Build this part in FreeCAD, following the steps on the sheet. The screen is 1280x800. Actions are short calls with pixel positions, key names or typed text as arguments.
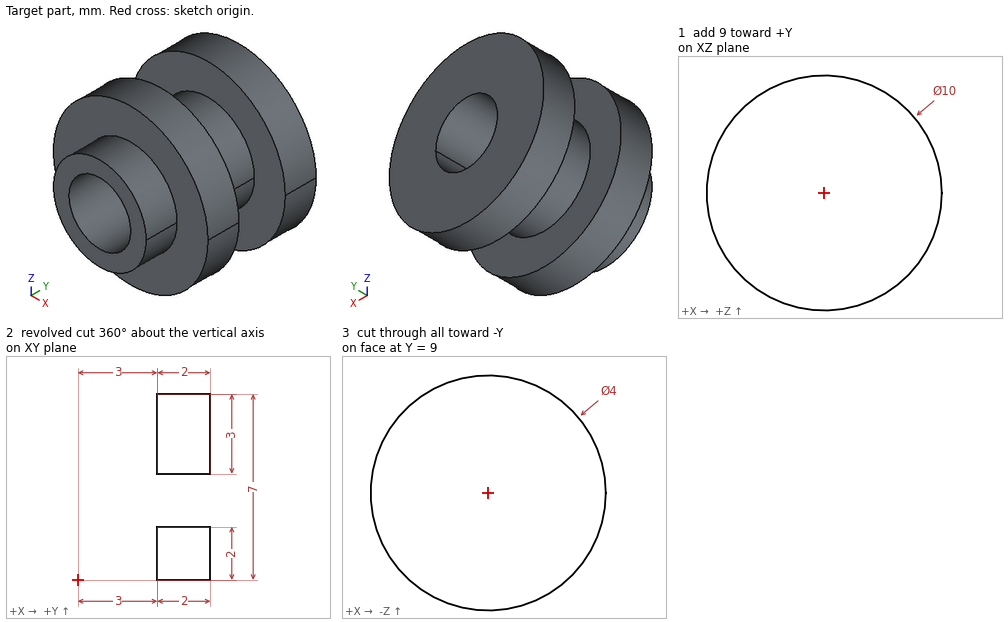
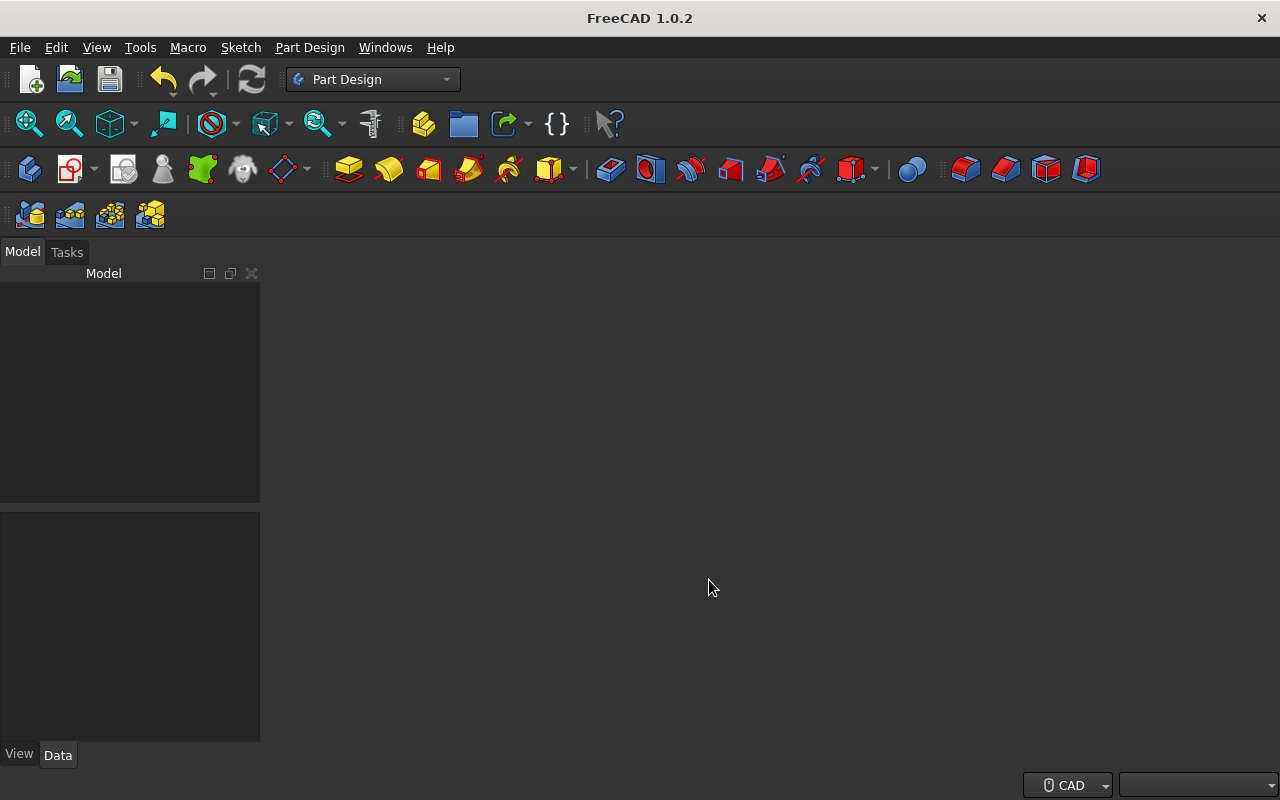
click(30, 80)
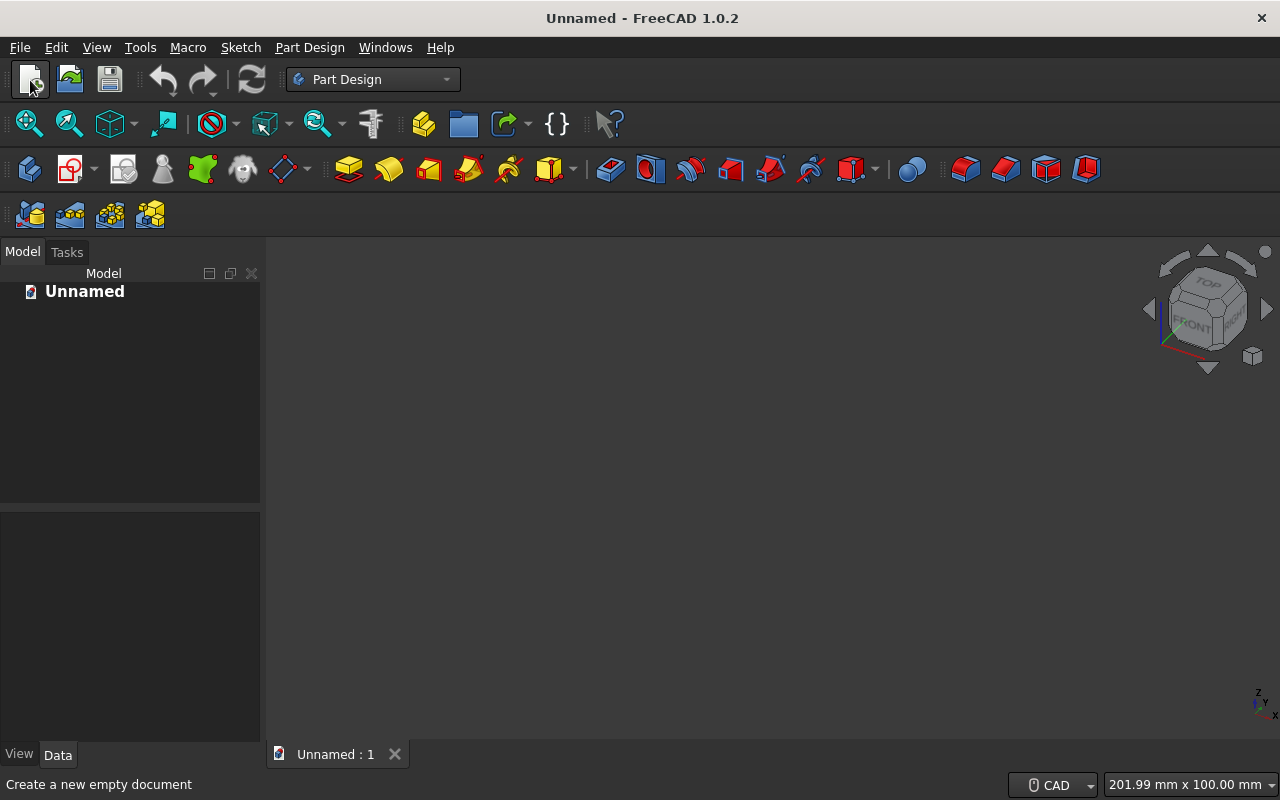
click(70, 170)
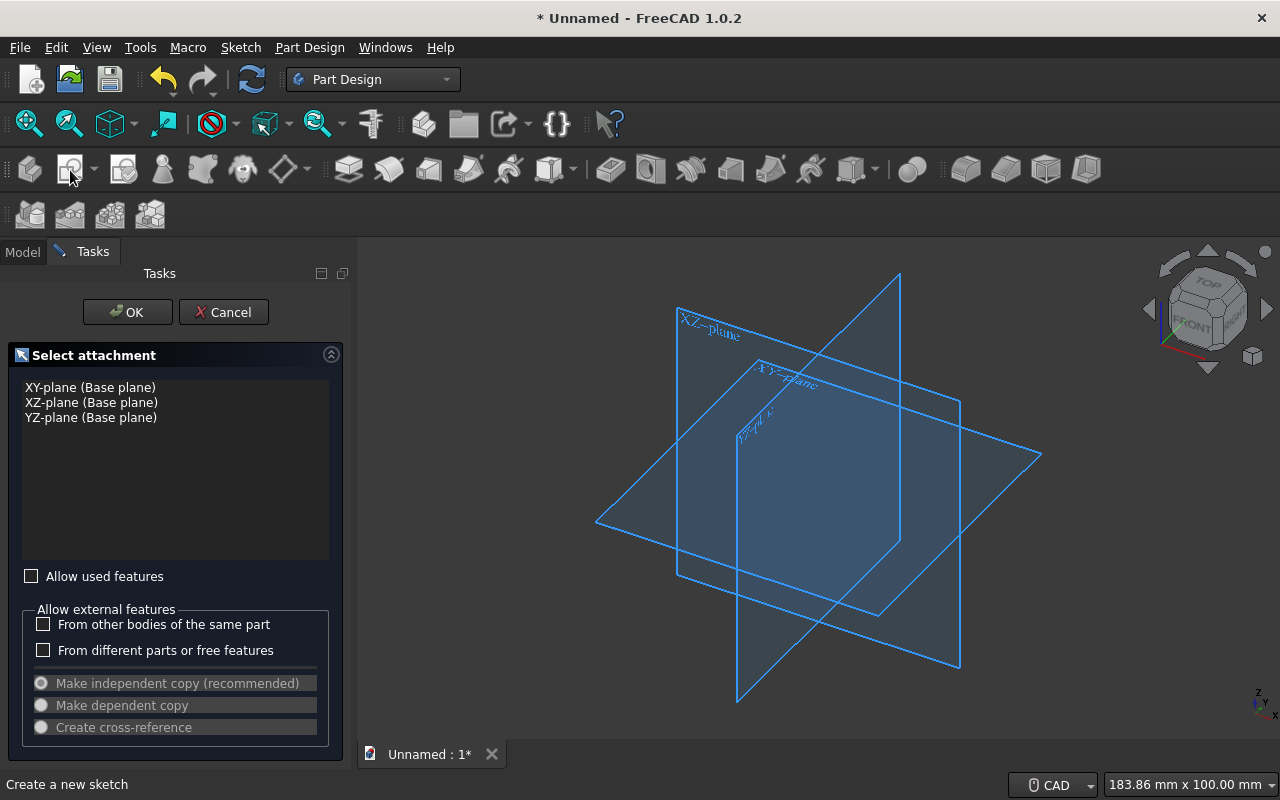
click(82, 402)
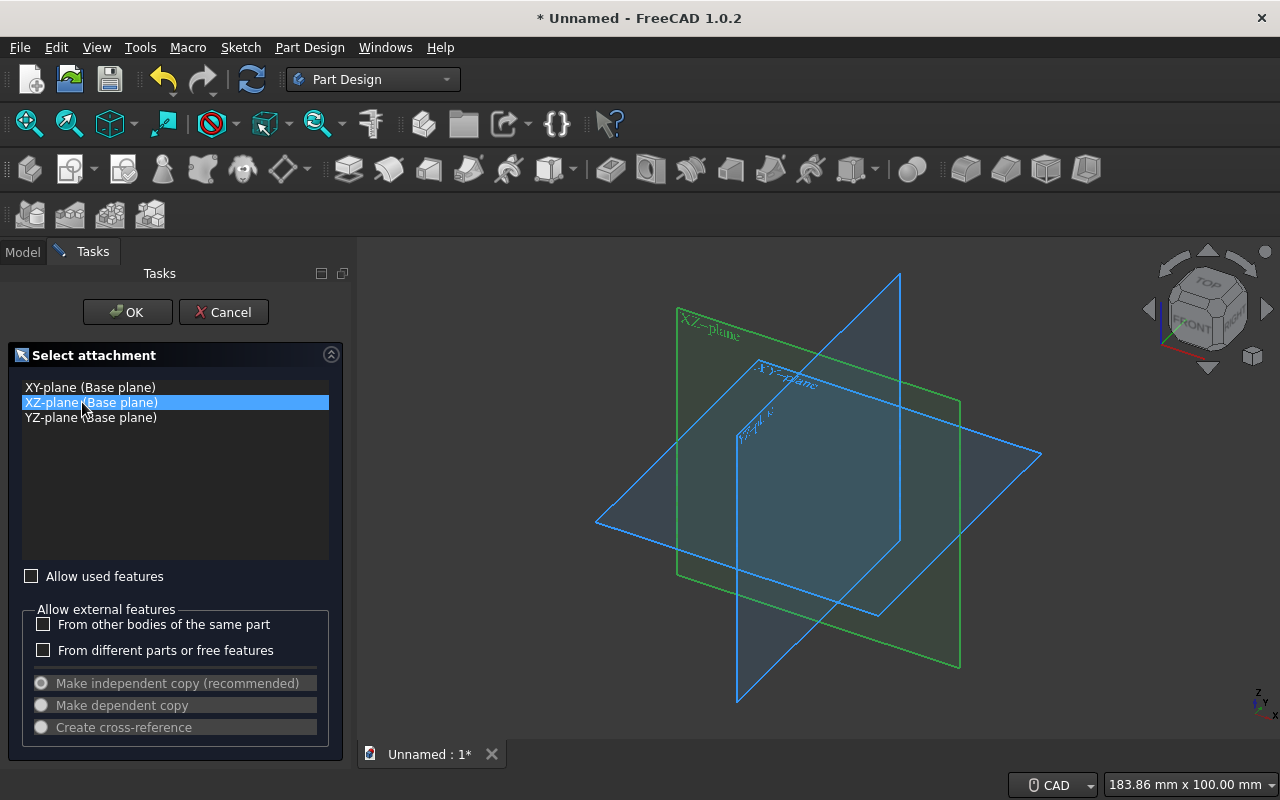
click(128, 312)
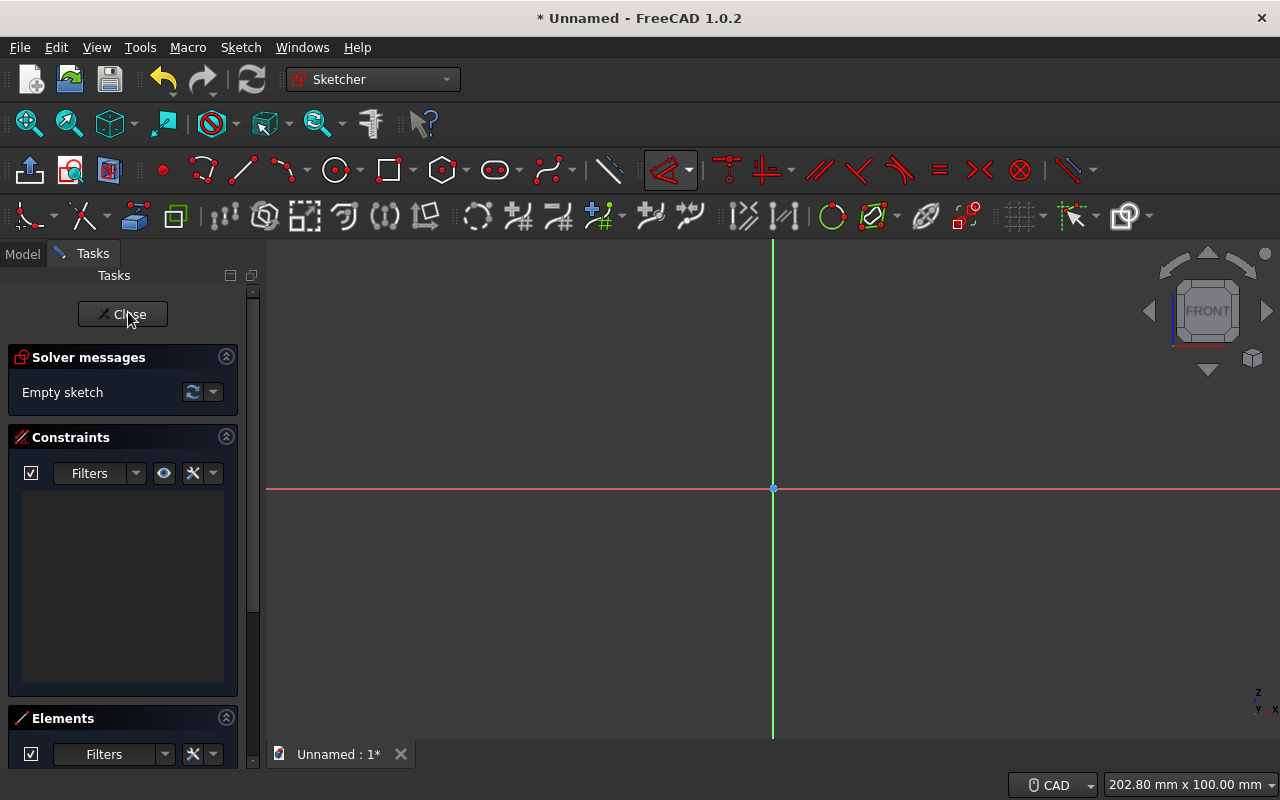
scroll(787, 489, up, 9)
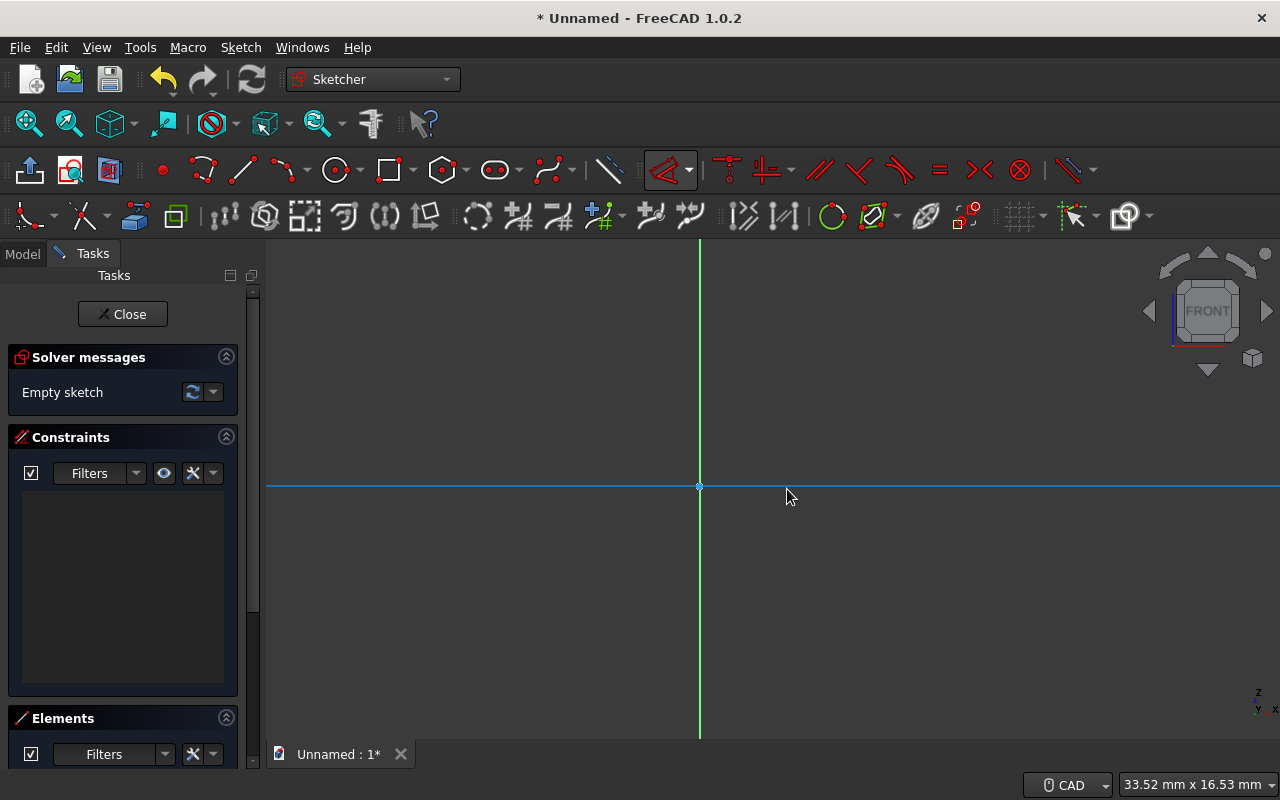
click(336, 170)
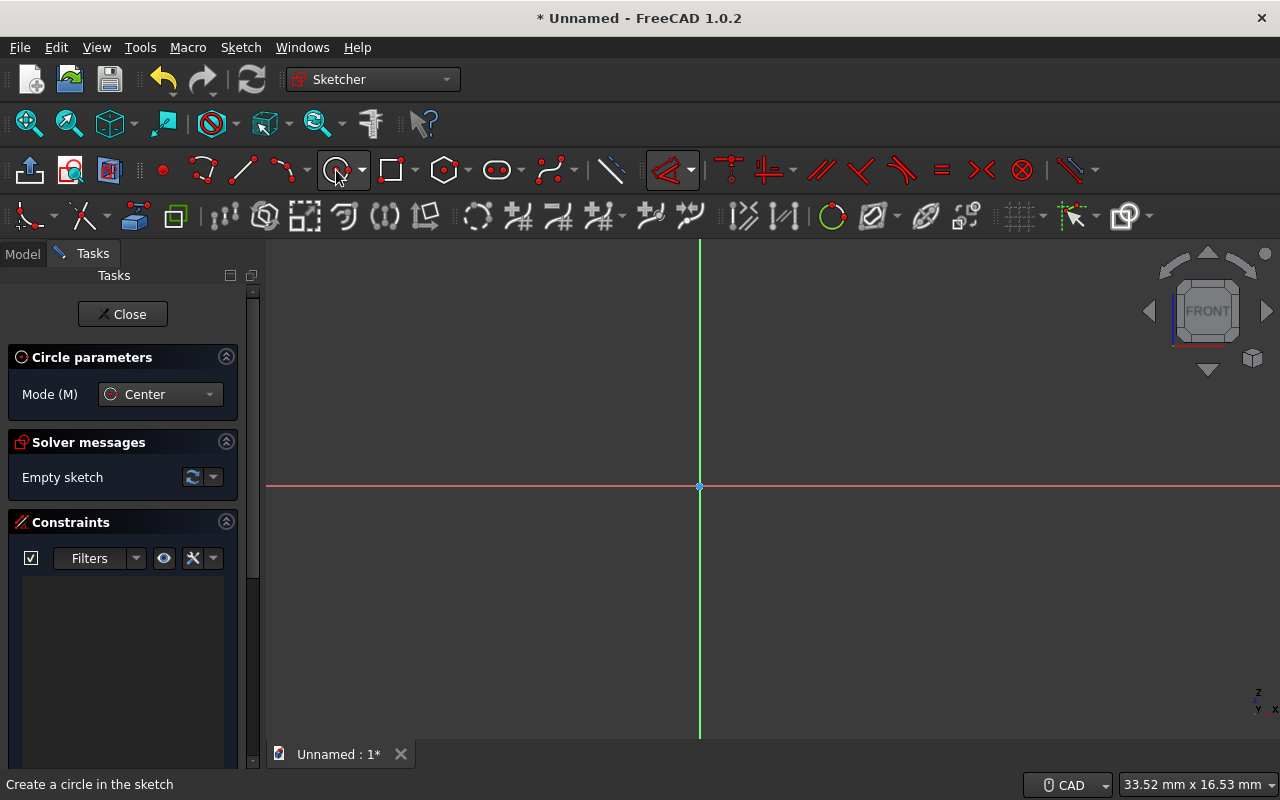
click(700, 486)
move(807, 380)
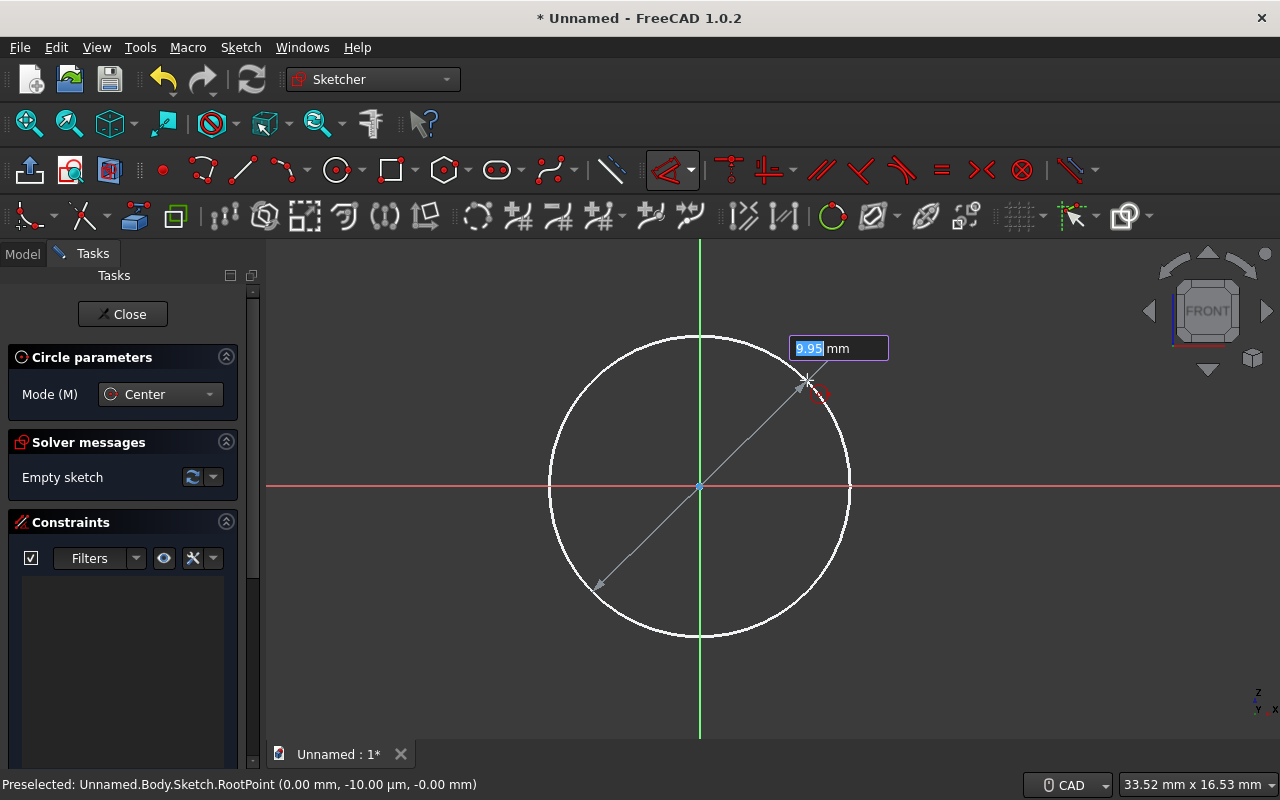
text(10)
key(Return)
key(Escape)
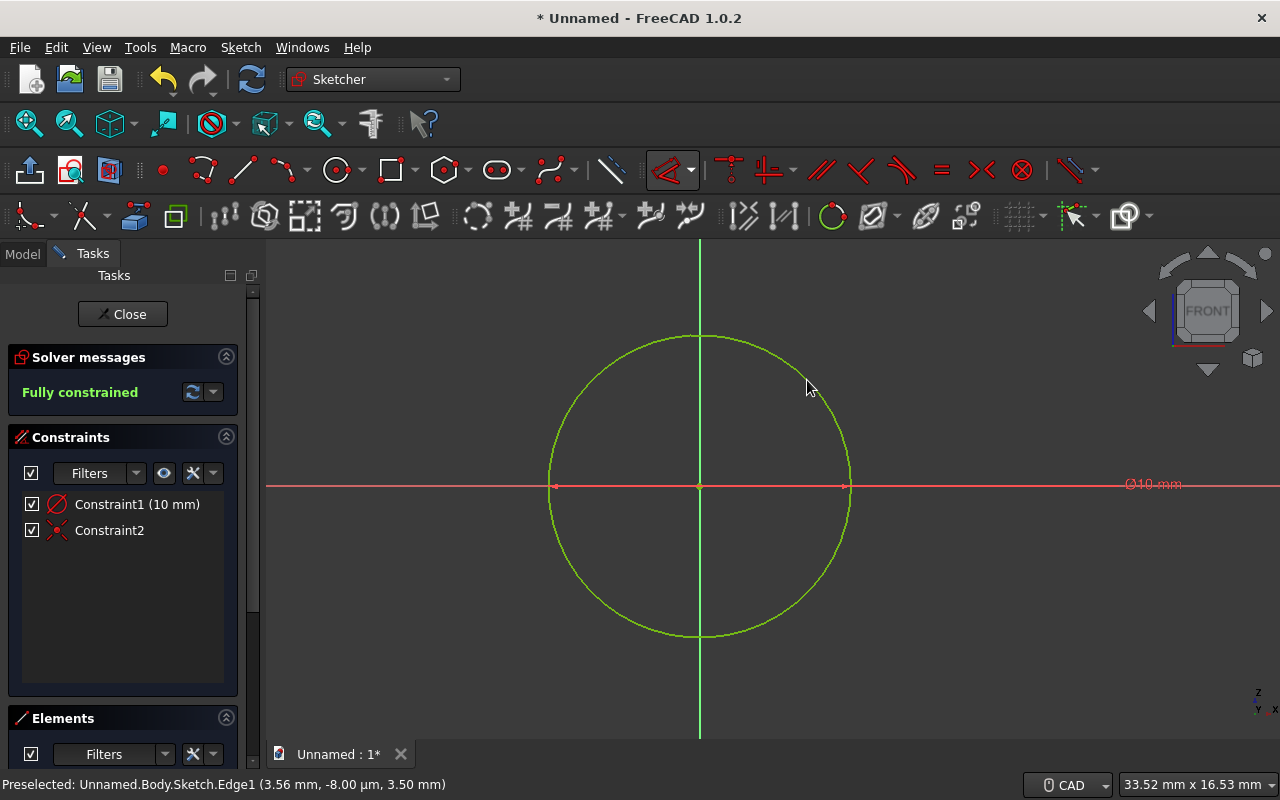
click(123, 314)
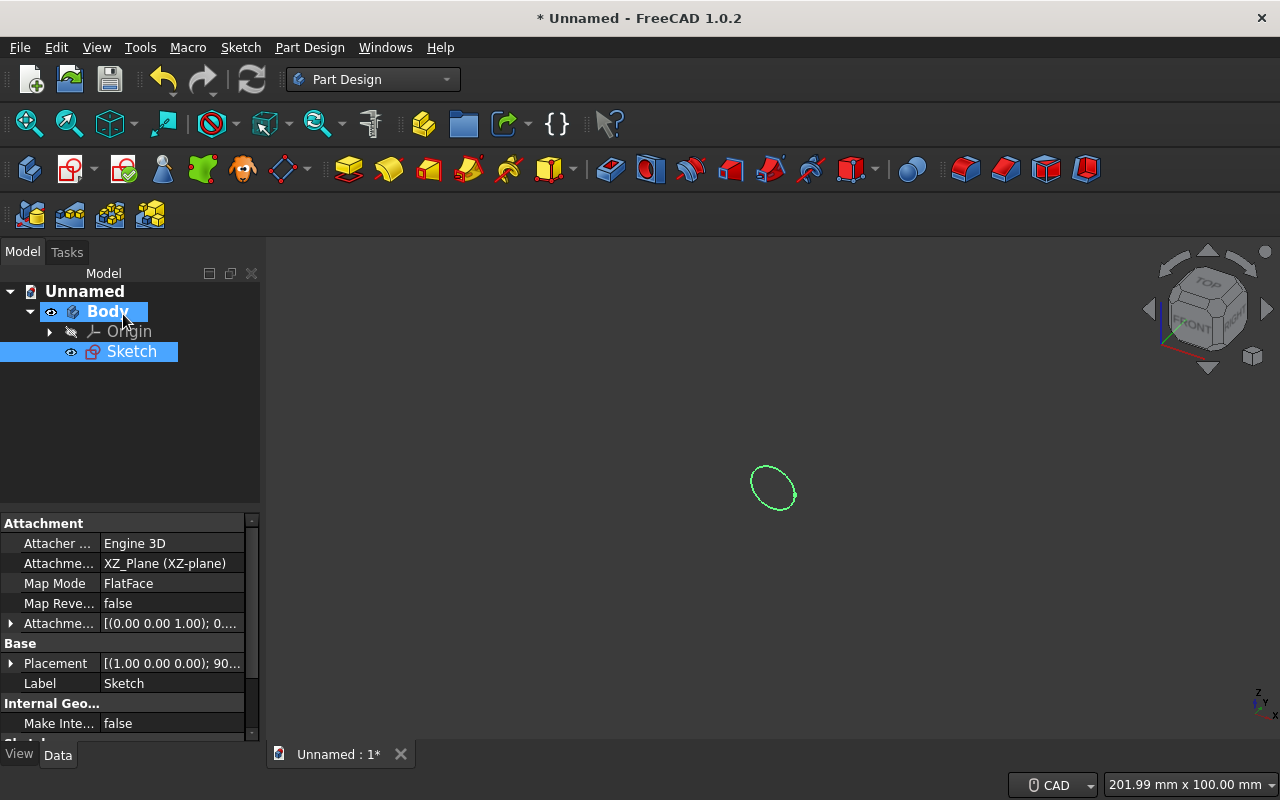
click(350, 170)